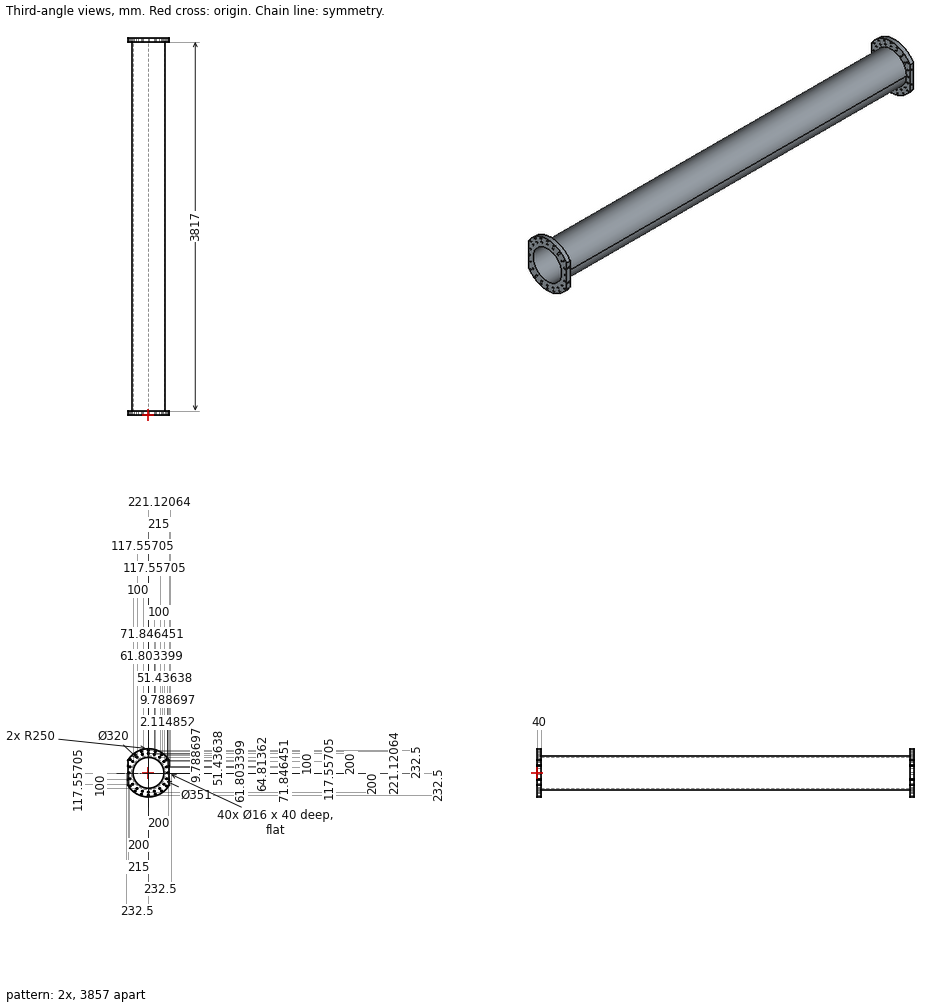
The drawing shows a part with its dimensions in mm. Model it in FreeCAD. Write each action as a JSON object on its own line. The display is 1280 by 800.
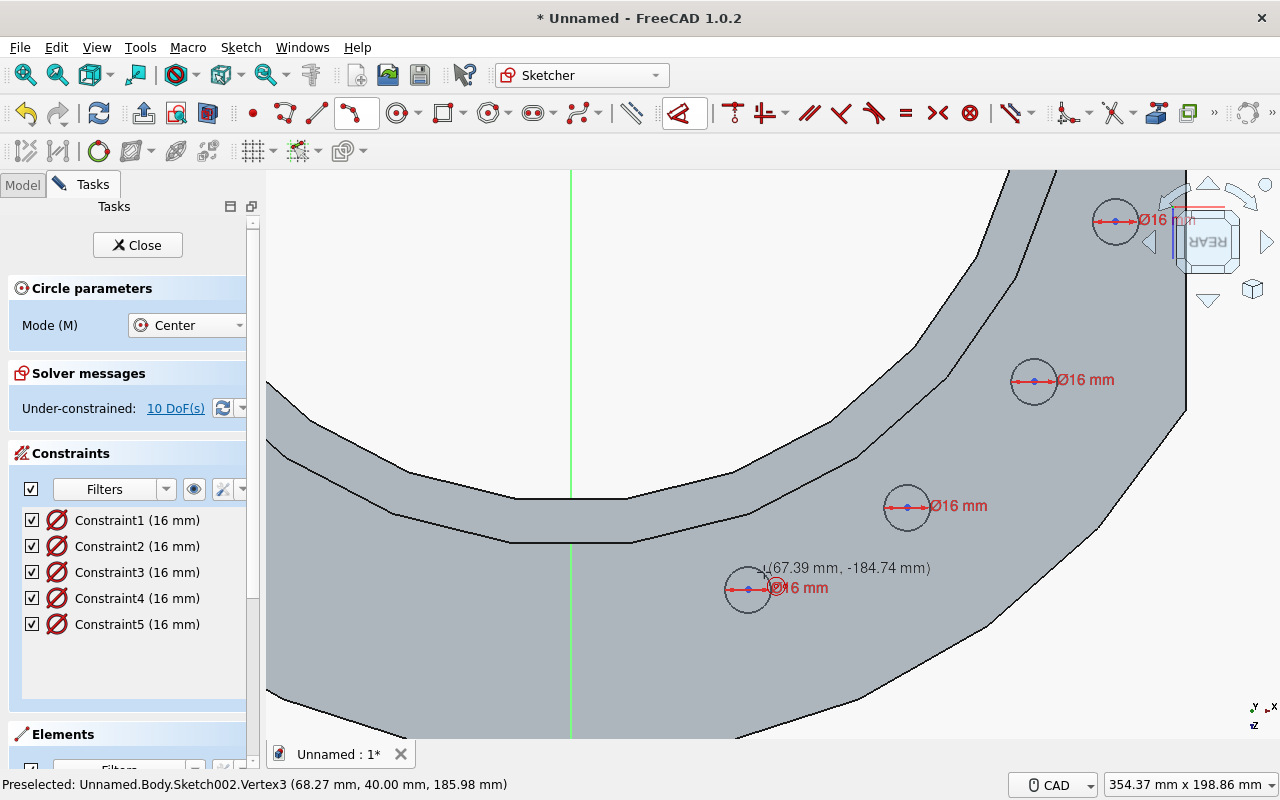
{"action": "left_click", "coordinate": [571, 617]}
{"action": "mouse_move", "coordinate": [587, 600]}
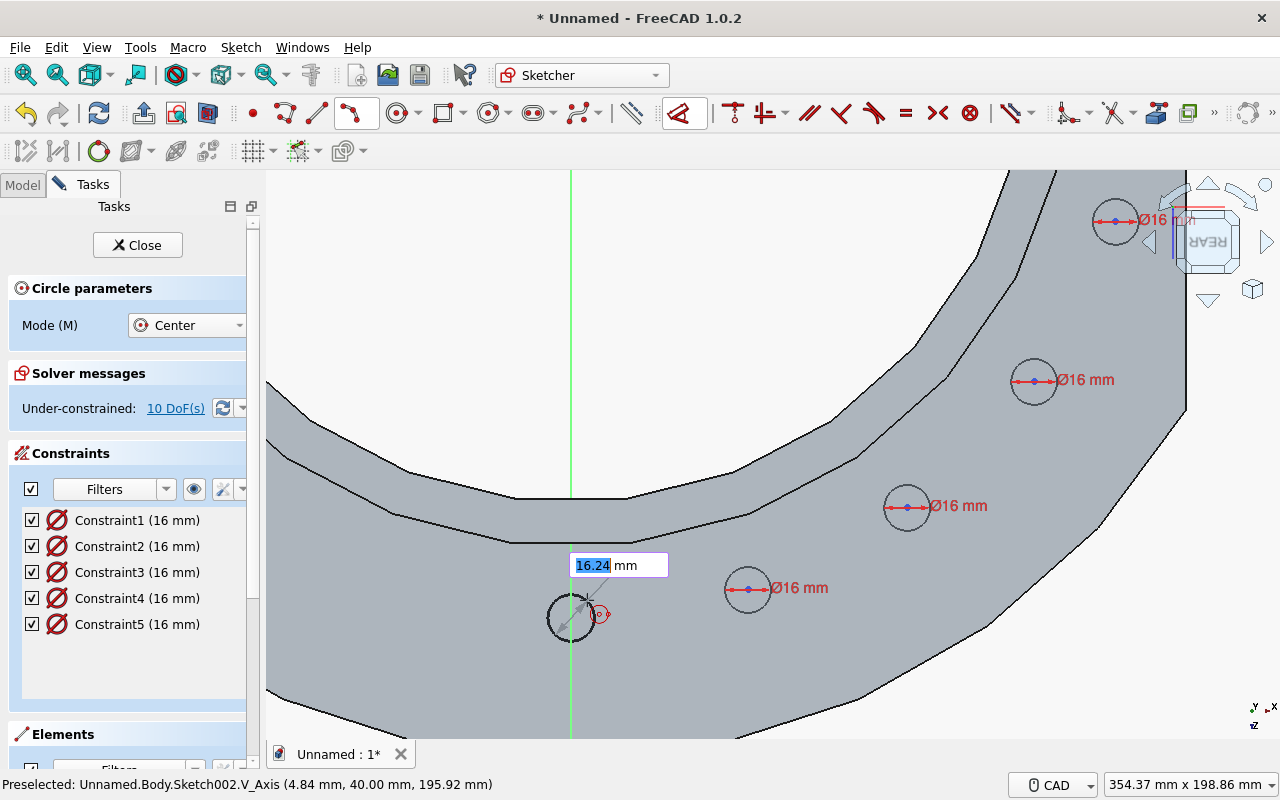
{"action": "type", "text": "16"}
{"action": "key", "text": "Return"}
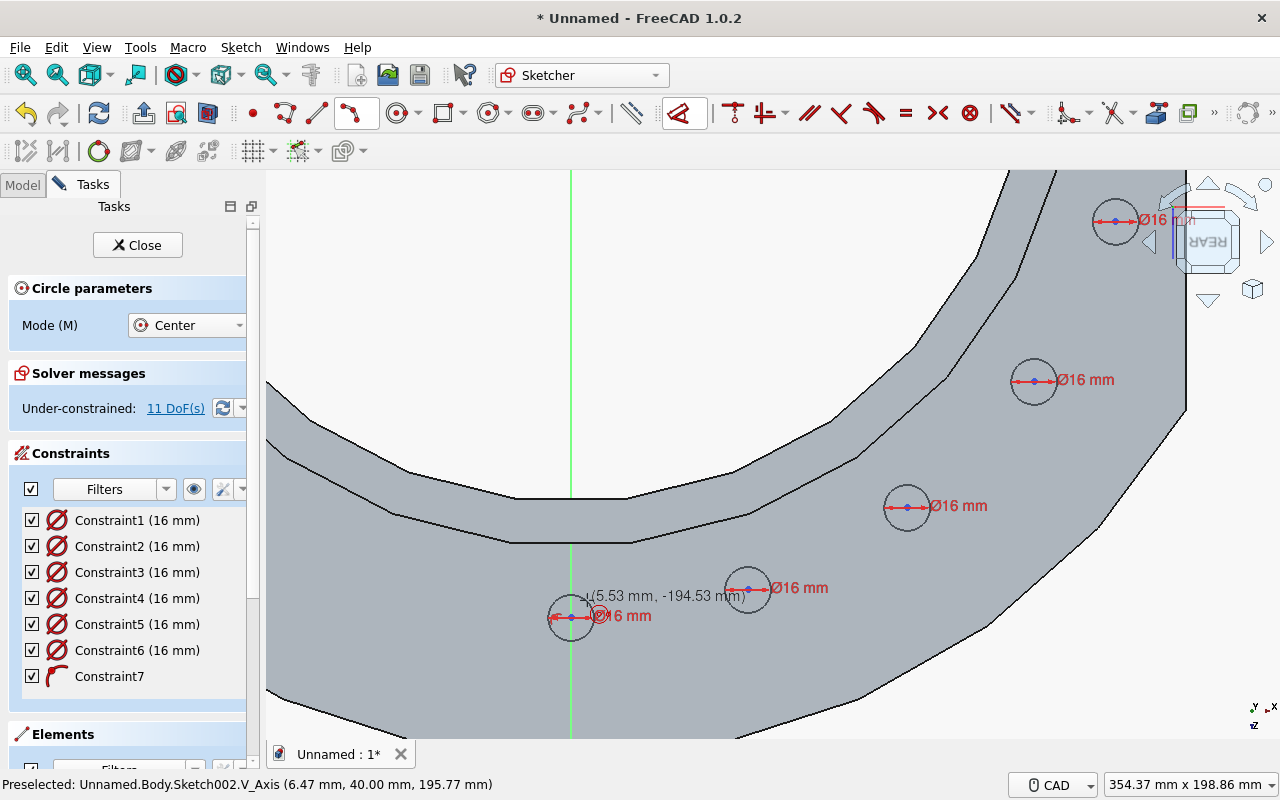
{"action": "left_click", "coordinate": [394, 589]}
{"action": "mouse_move", "coordinate": [411, 572]}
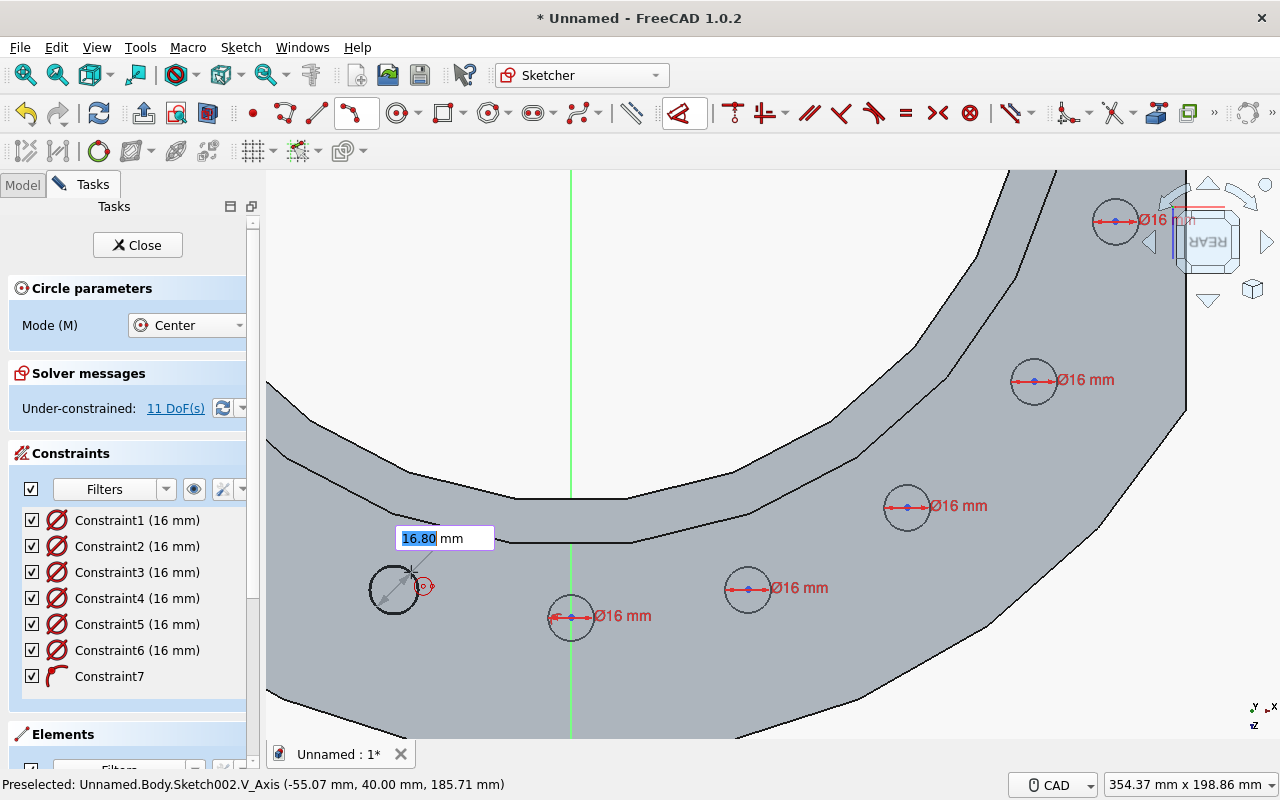
{"action": "type", "text": "16"}
{"action": "key", "text": "Return"}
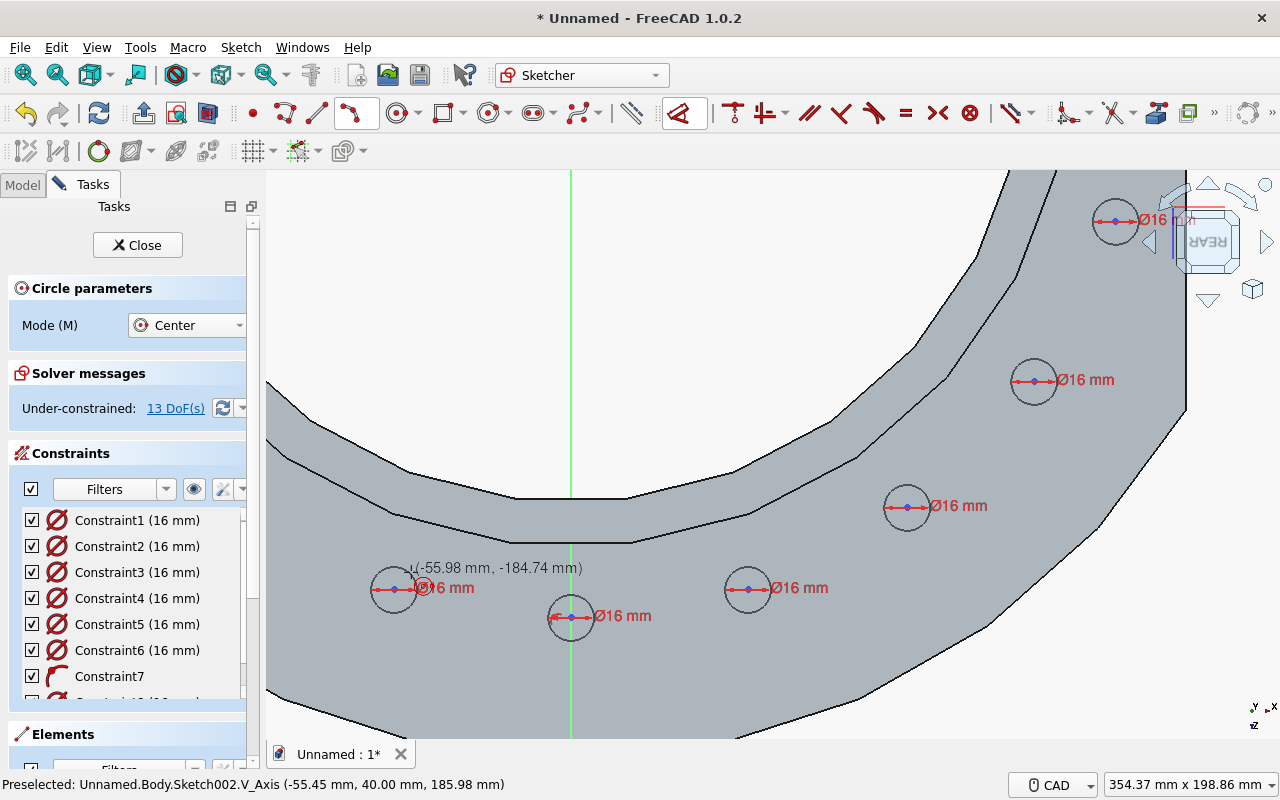
{"action": "scroll", "coordinate": [748, 589], "scroll_direction": "down", "scroll_amount": 7}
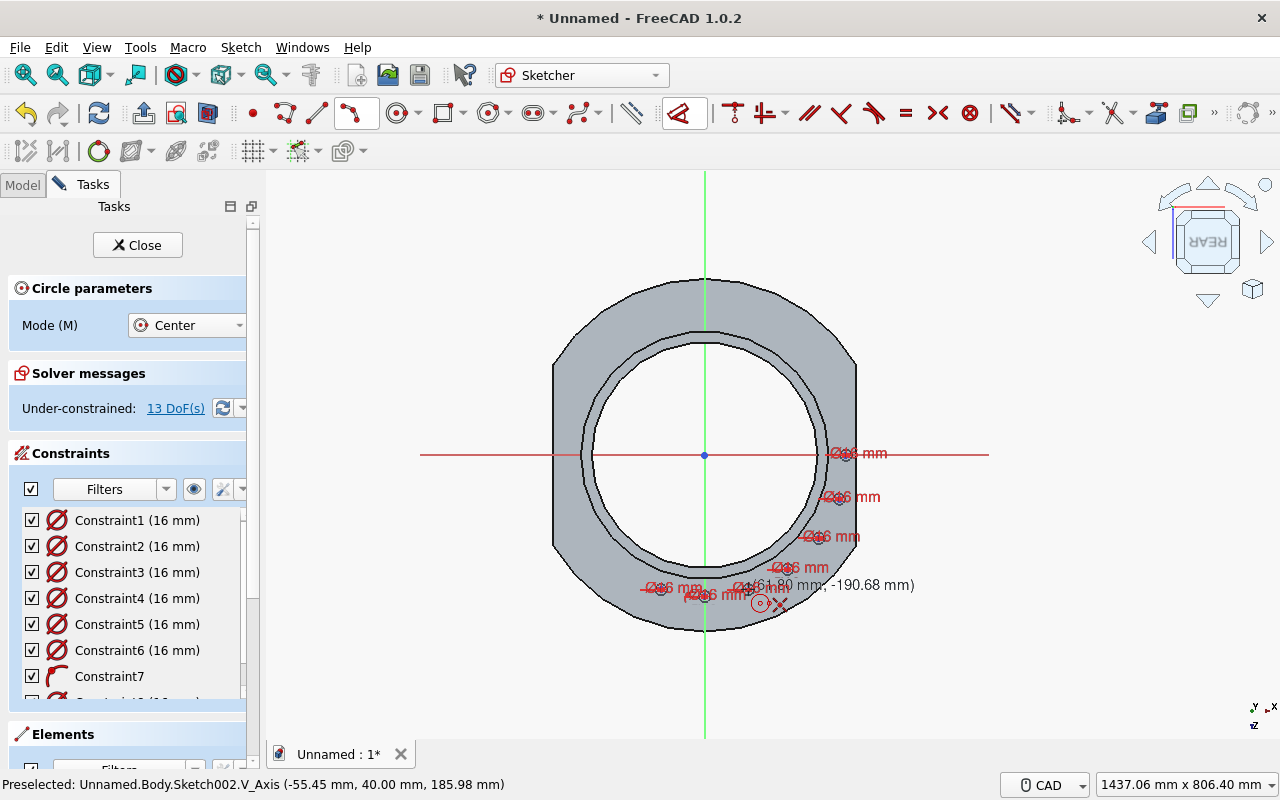
{"action": "scroll", "coordinate": [622, 569], "scroll_direction": "up", "scroll_amount": 7}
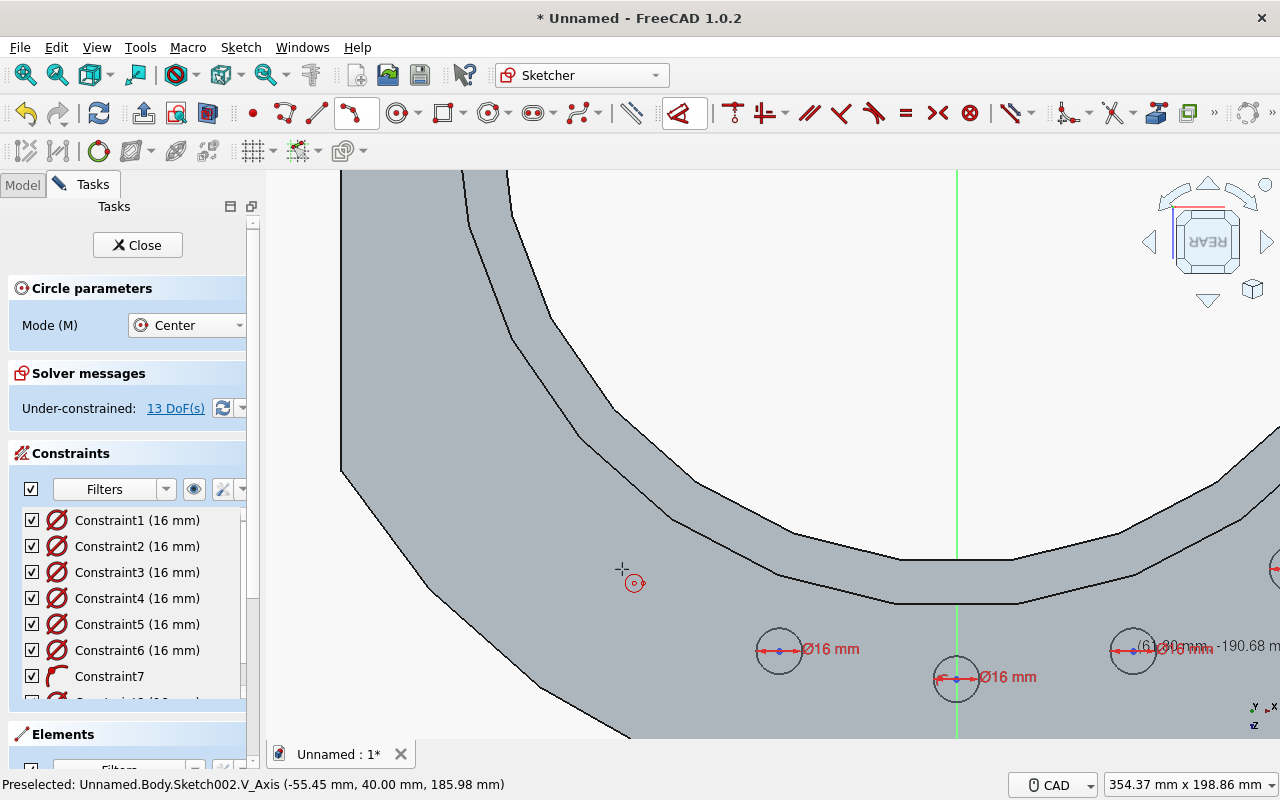
{"action": "left_click", "coordinate": [620, 569]}
{"action": "mouse_move", "coordinate": [636, 552]}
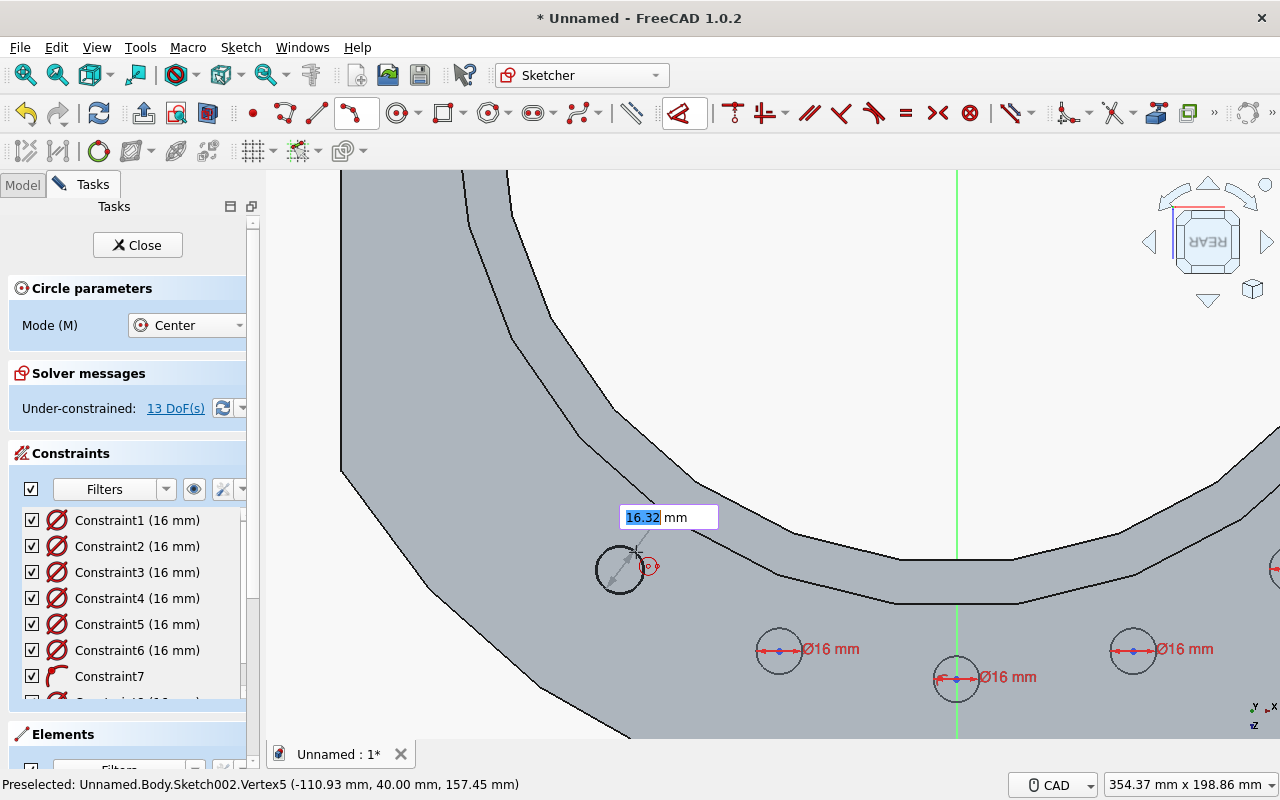
{"action": "type", "text": "16"}
{"action": "key", "text": "Return"}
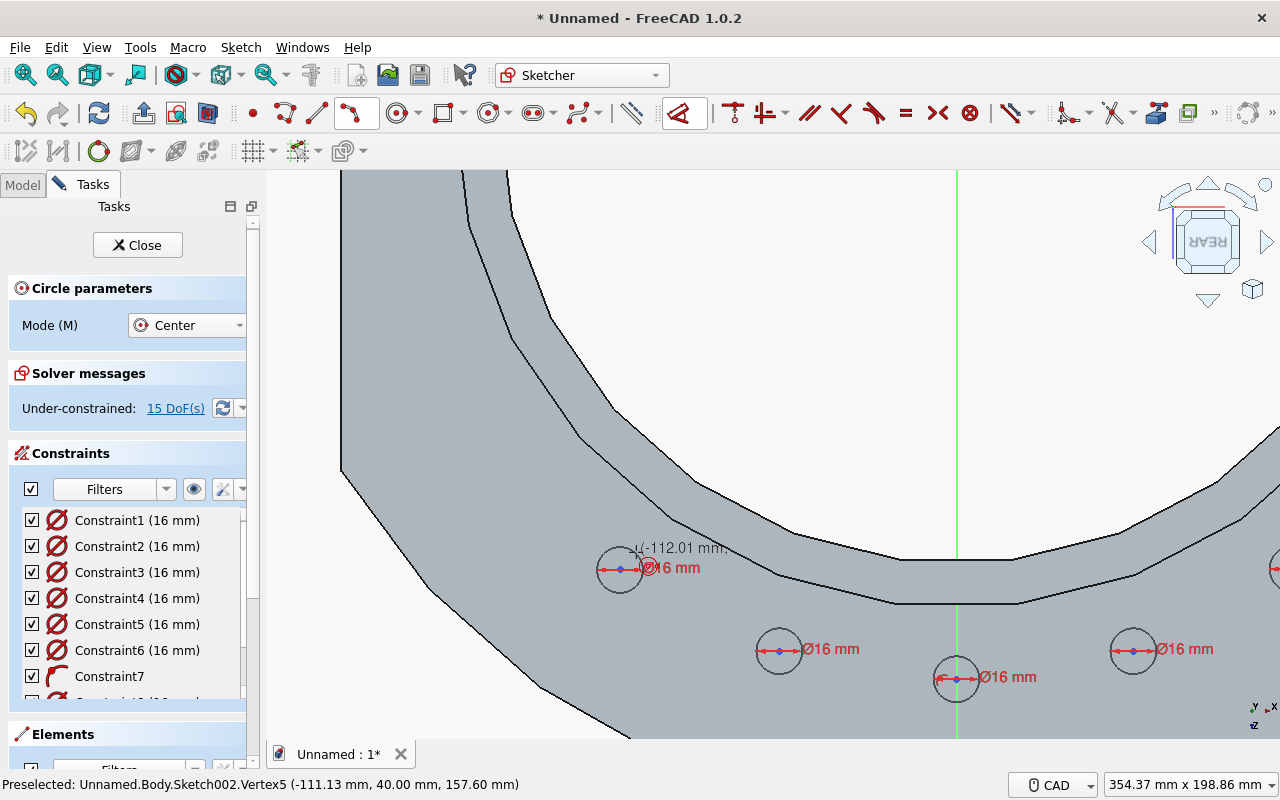
{"action": "left_click", "coordinate": [494, 442]}
{"action": "mouse_move", "coordinate": [510, 426]}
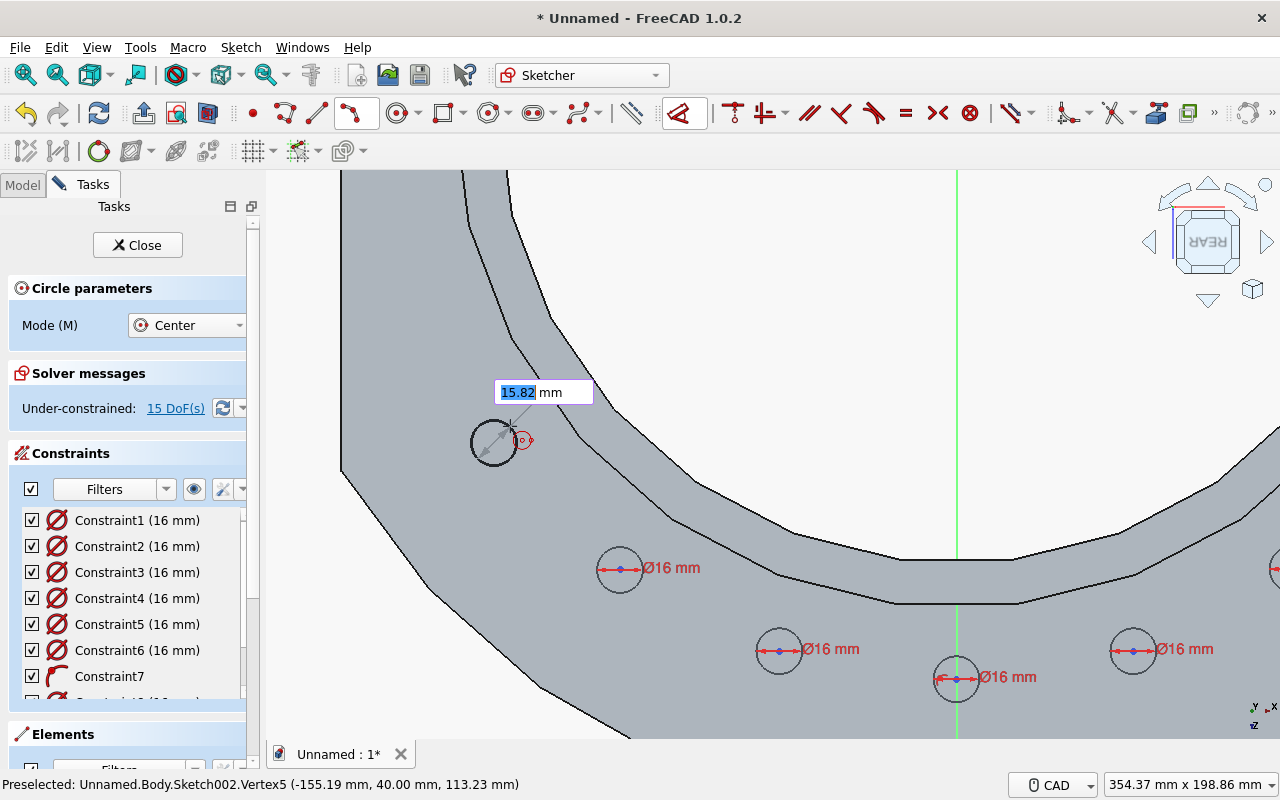
{"action": "type", "text": "16"}
{"action": "key", "text": "Return"}